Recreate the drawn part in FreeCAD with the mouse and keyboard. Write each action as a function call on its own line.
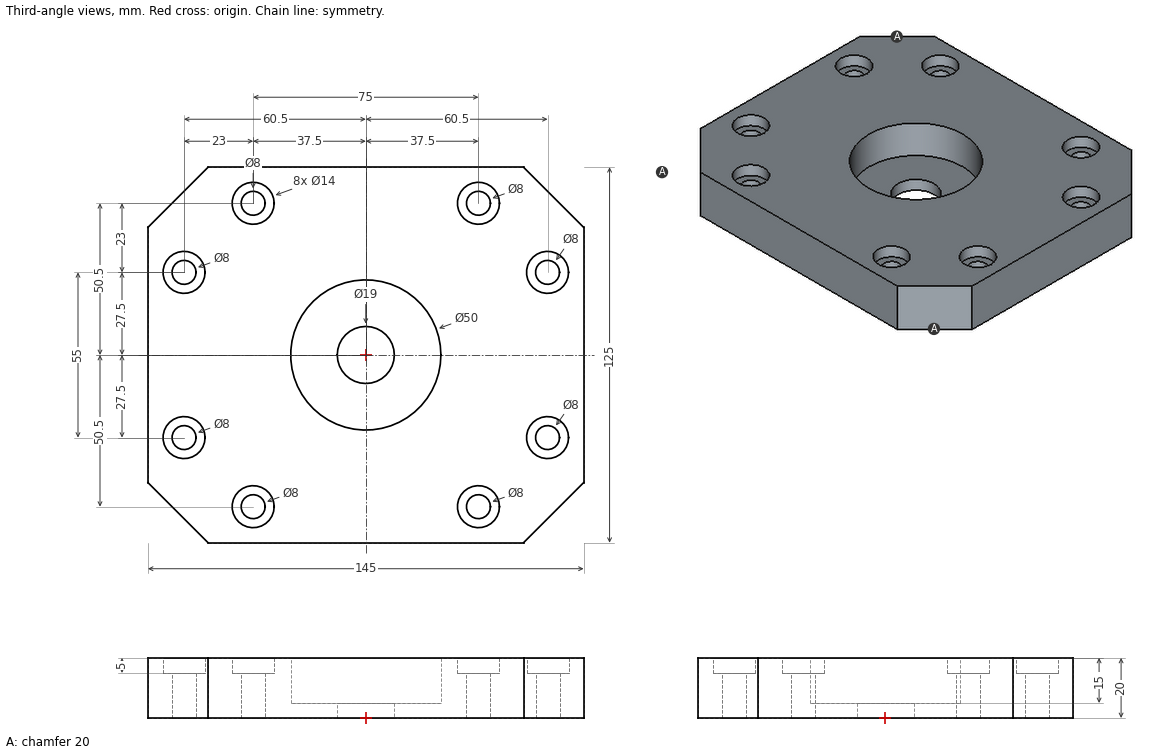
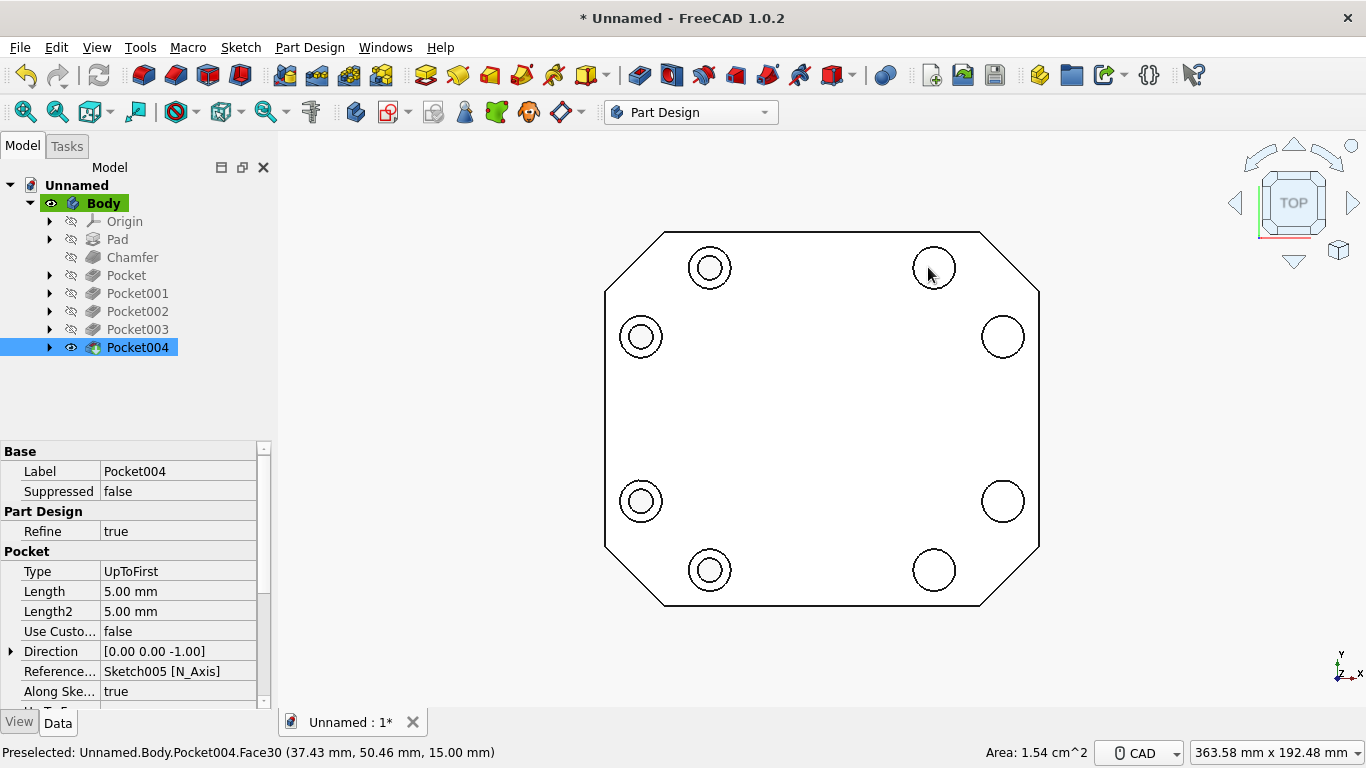
click(388, 112)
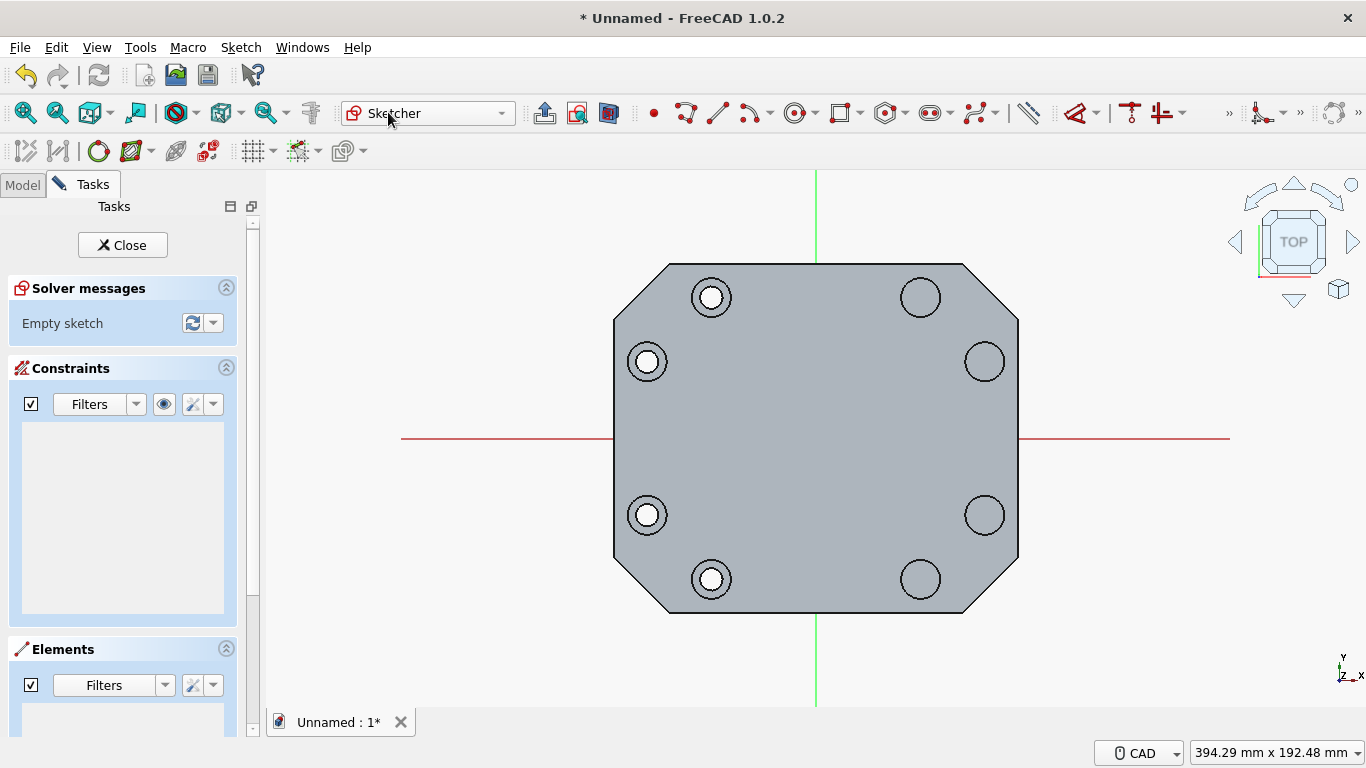
scroll(932, 288, up, 14)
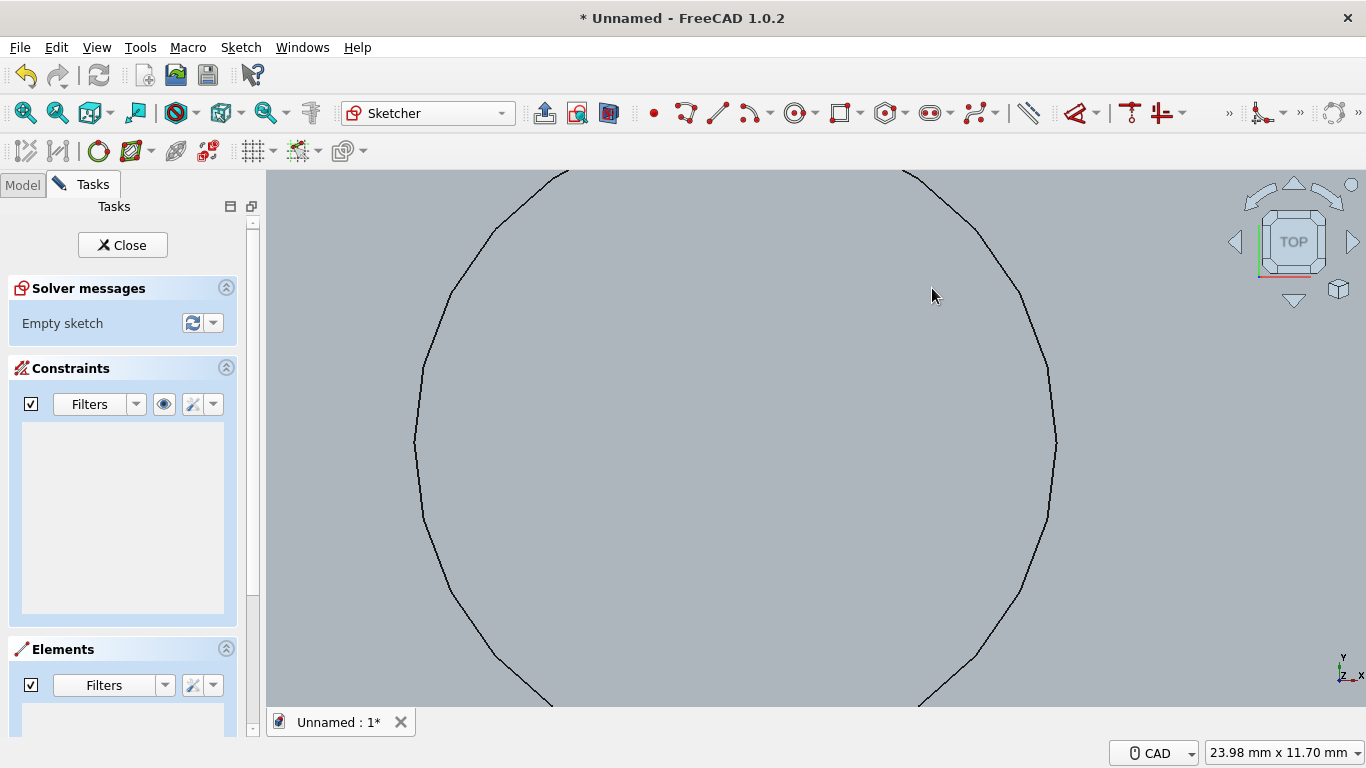
click(796, 114)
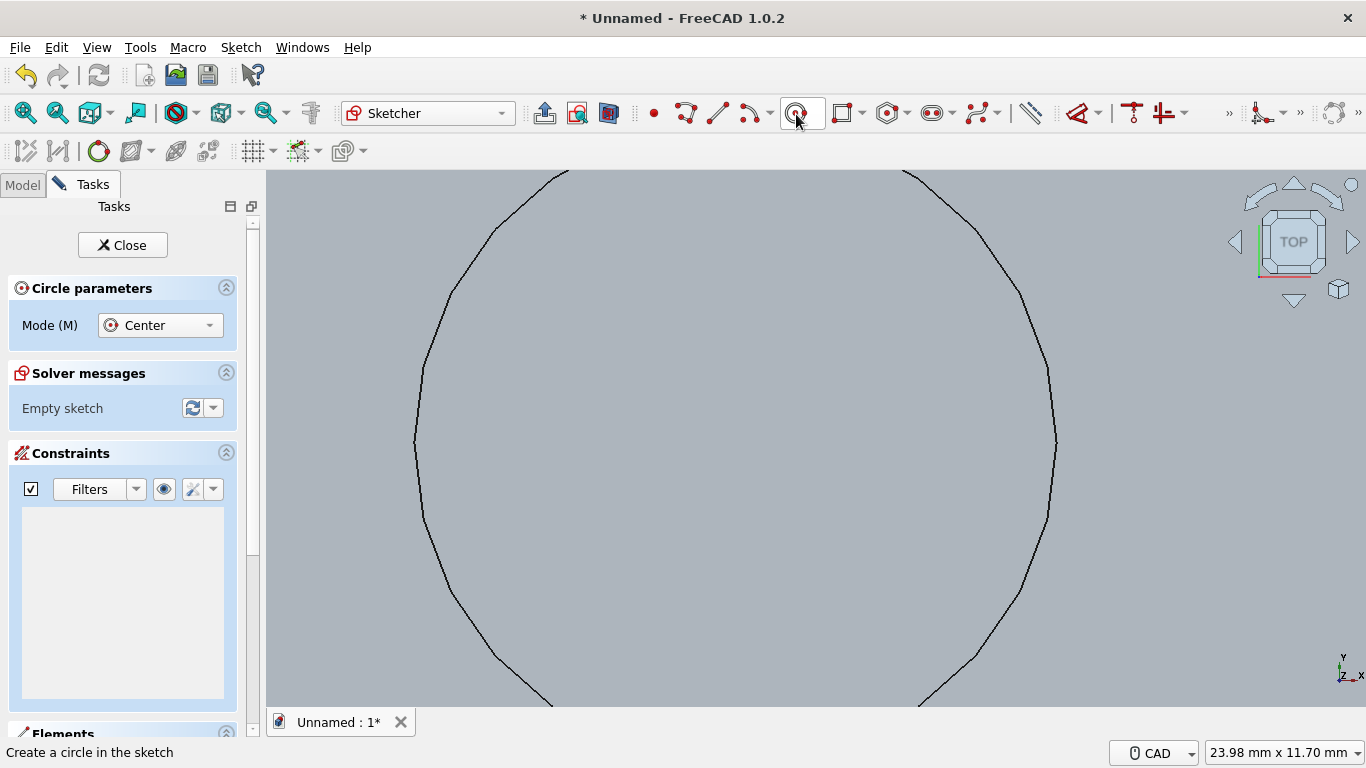
click(735, 443)
click(865, 313)
key(Escape)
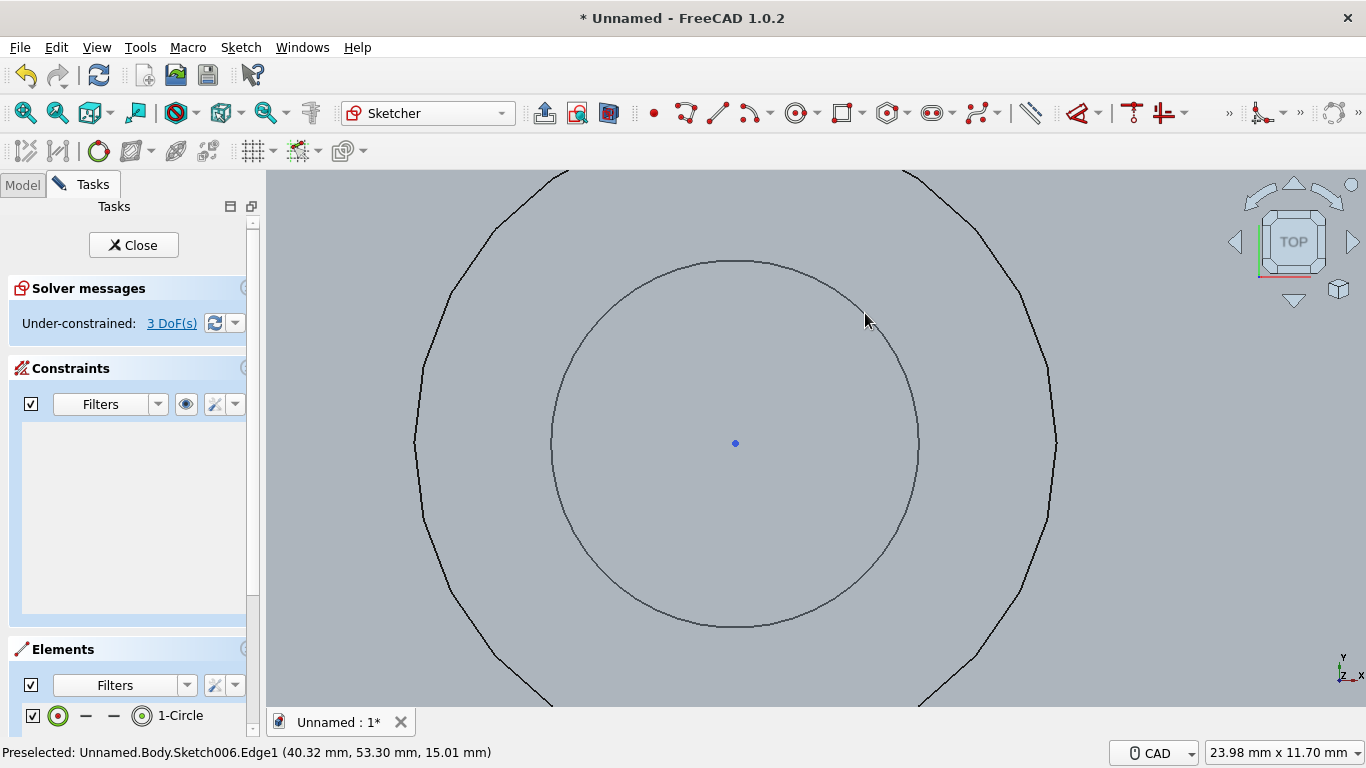
key(d)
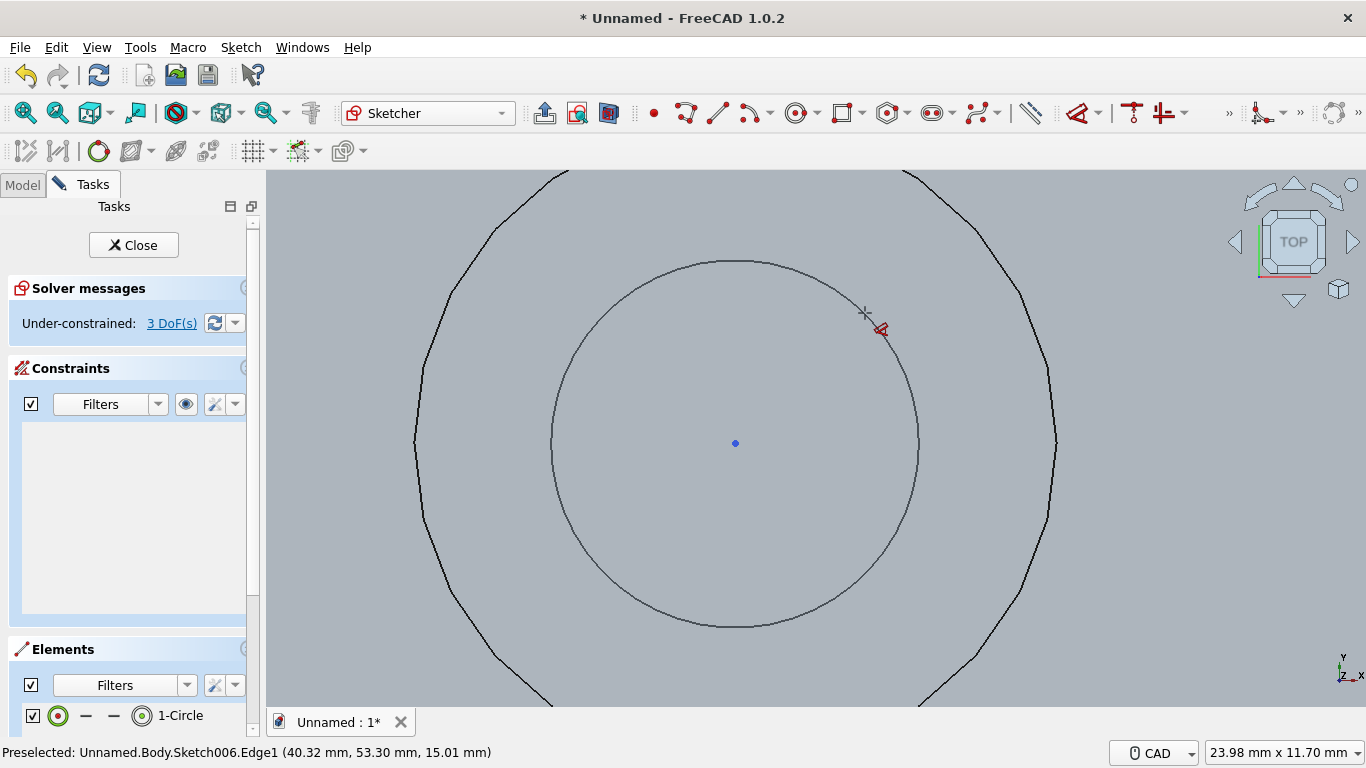
click(865, 314)
click(888, 291)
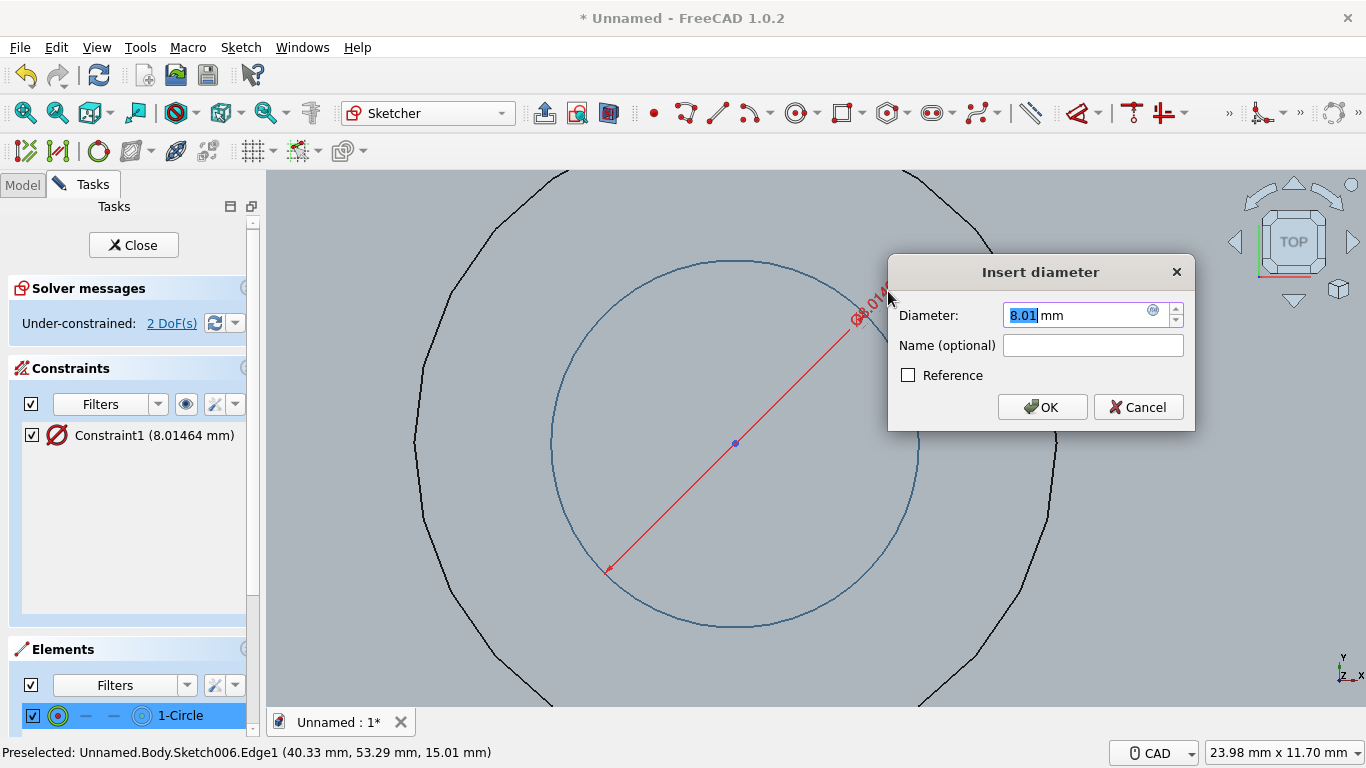
text(8)
key(Return)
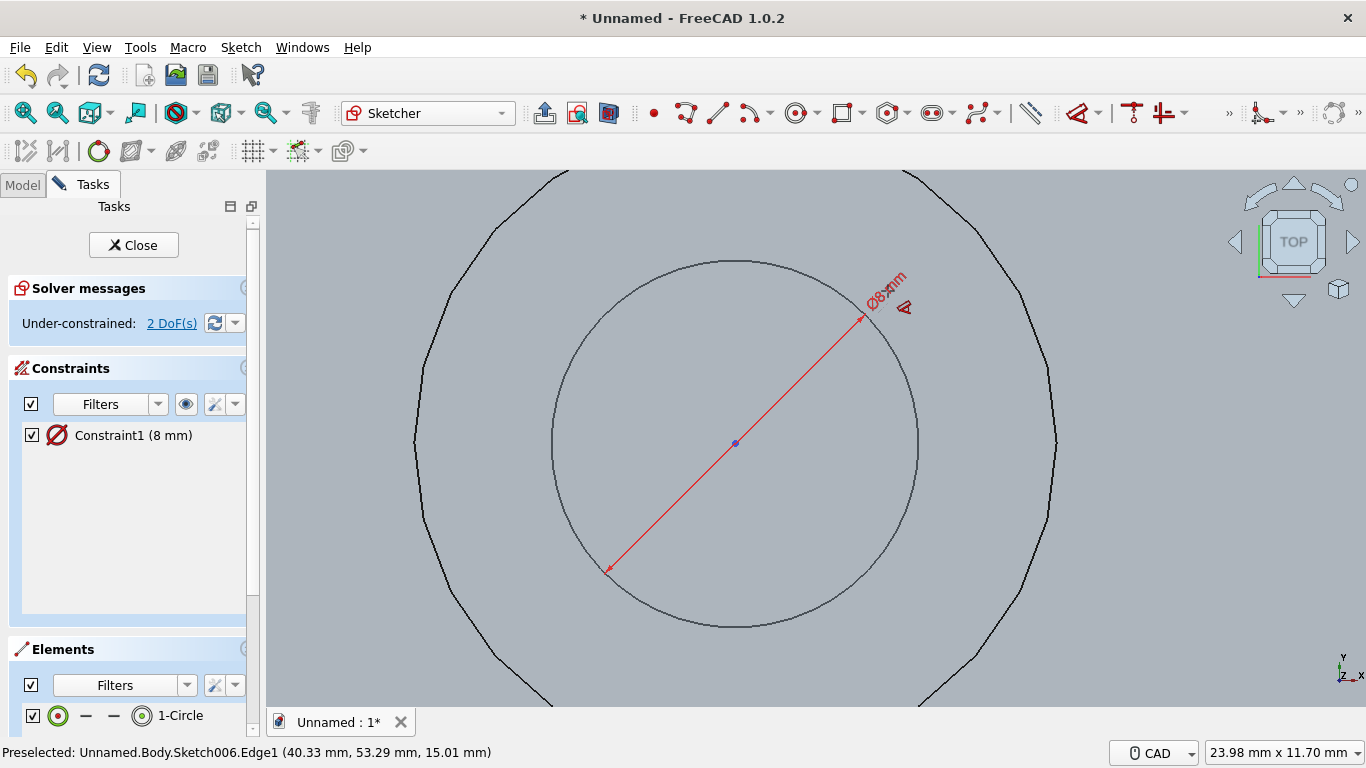
click(735, 444)
click(514, 410)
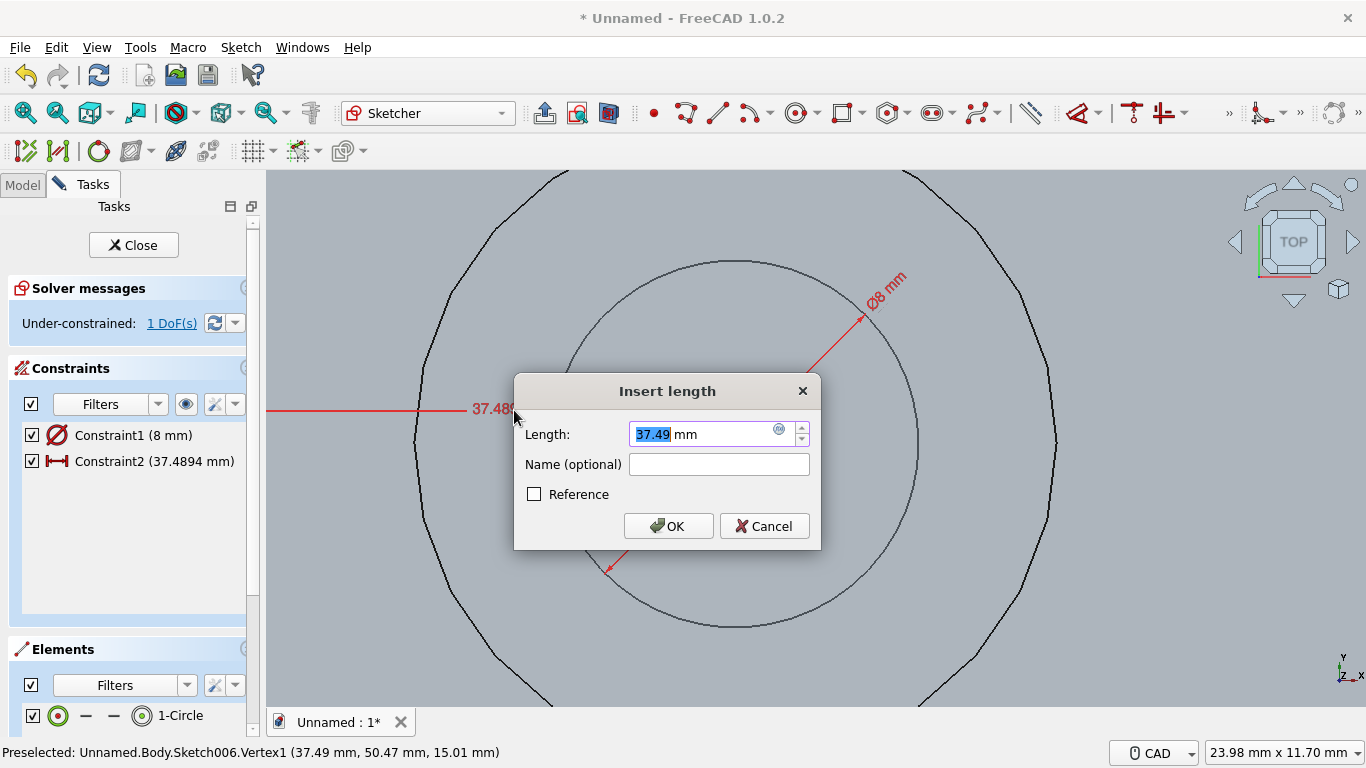
text(37.5)
key(Return)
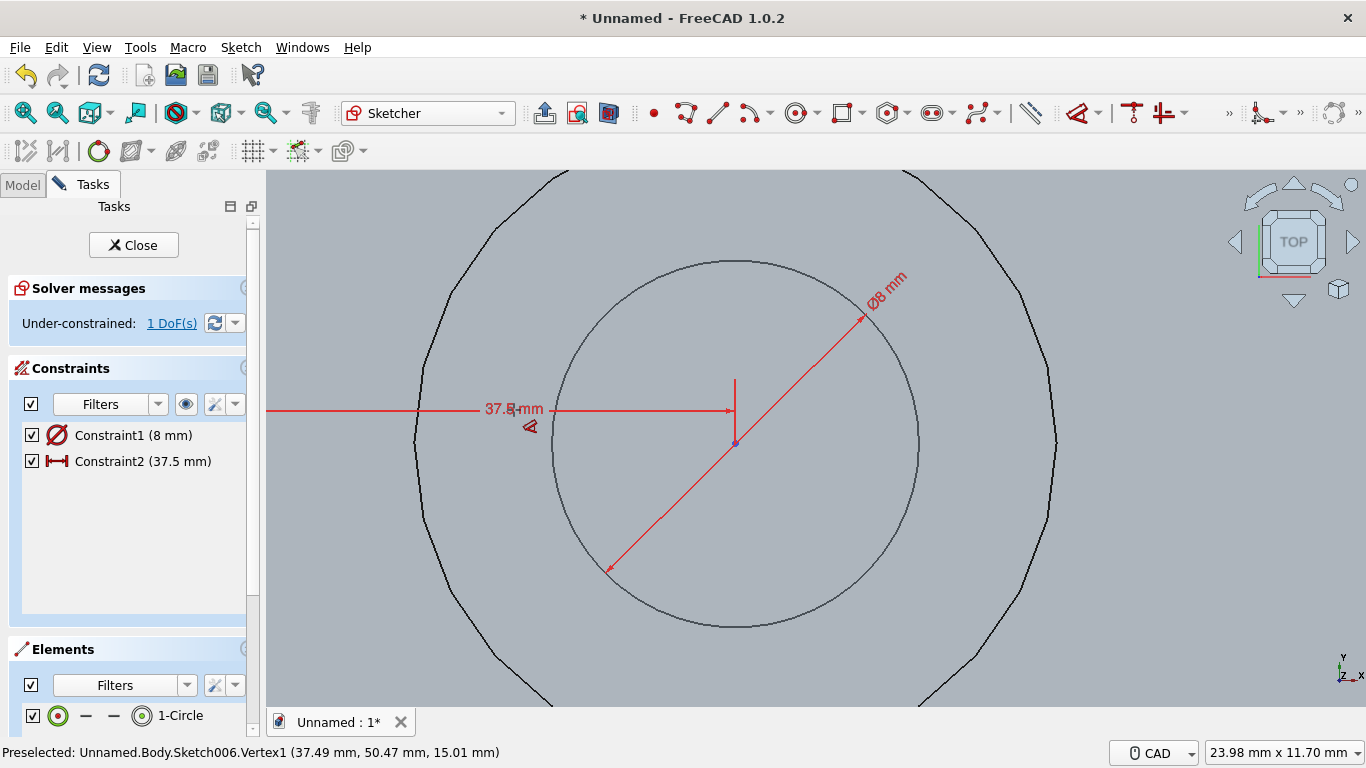
click(735, 444)
click(769, 562)